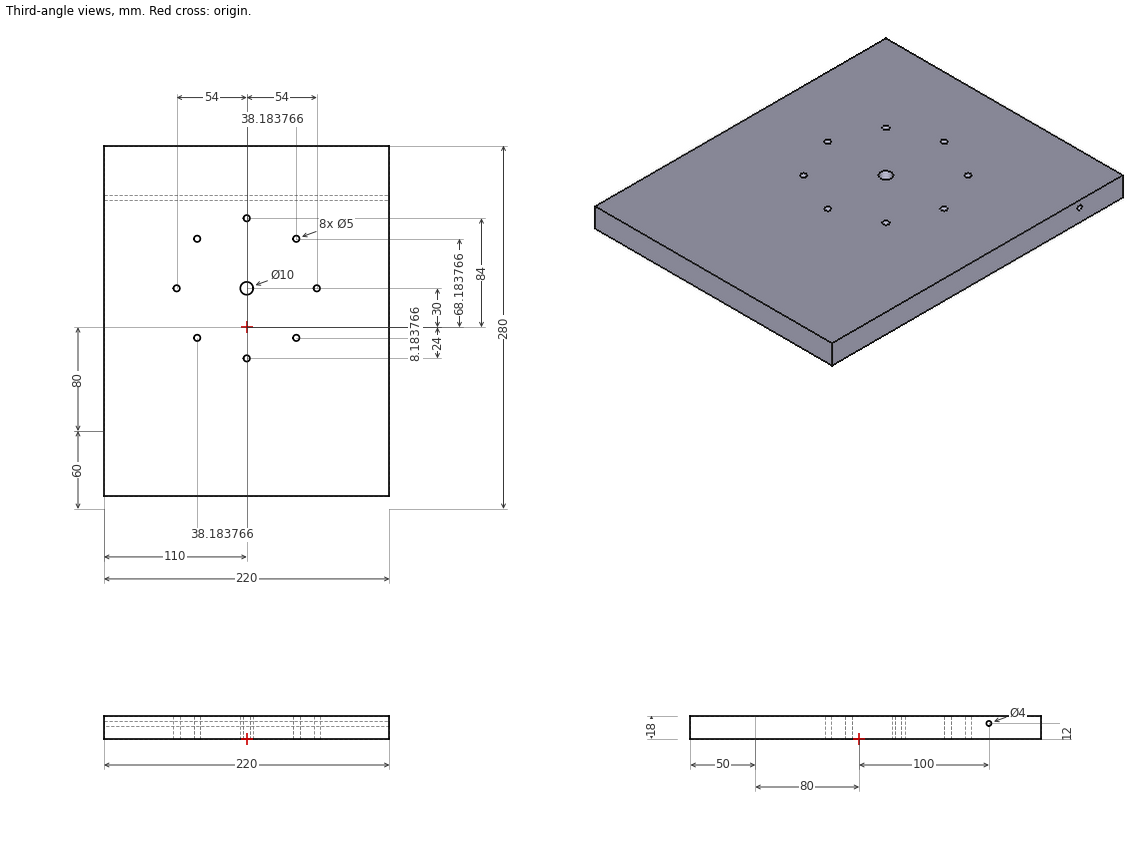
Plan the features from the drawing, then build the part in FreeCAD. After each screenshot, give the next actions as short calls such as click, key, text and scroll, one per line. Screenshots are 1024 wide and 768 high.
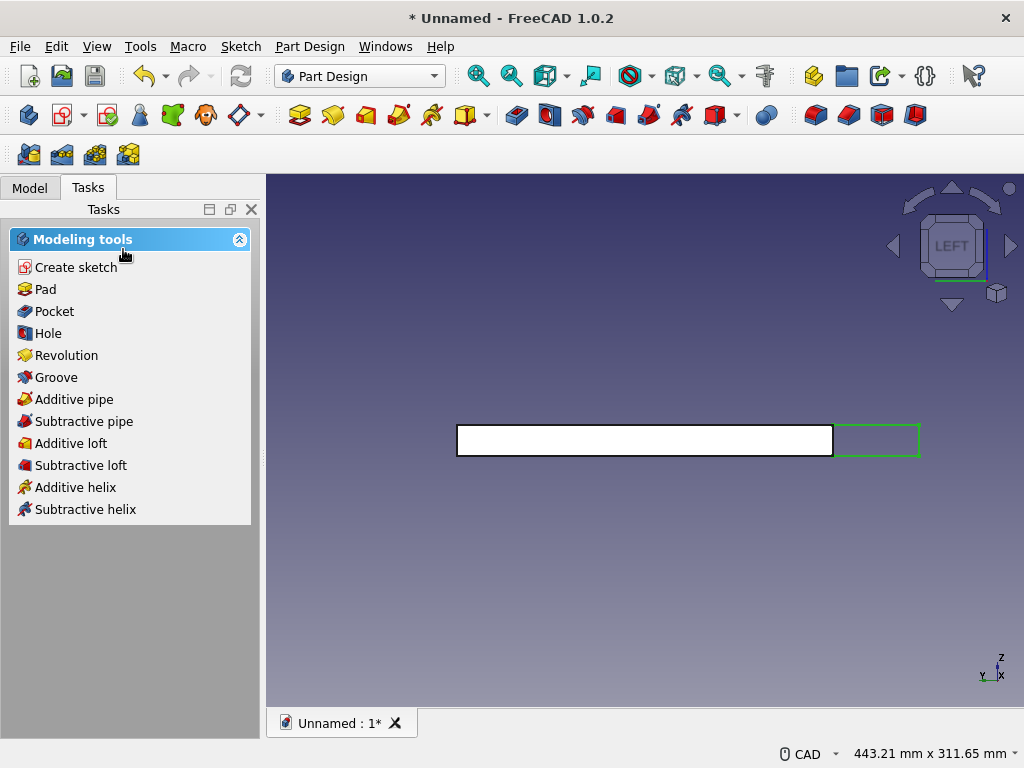
click(300, 116)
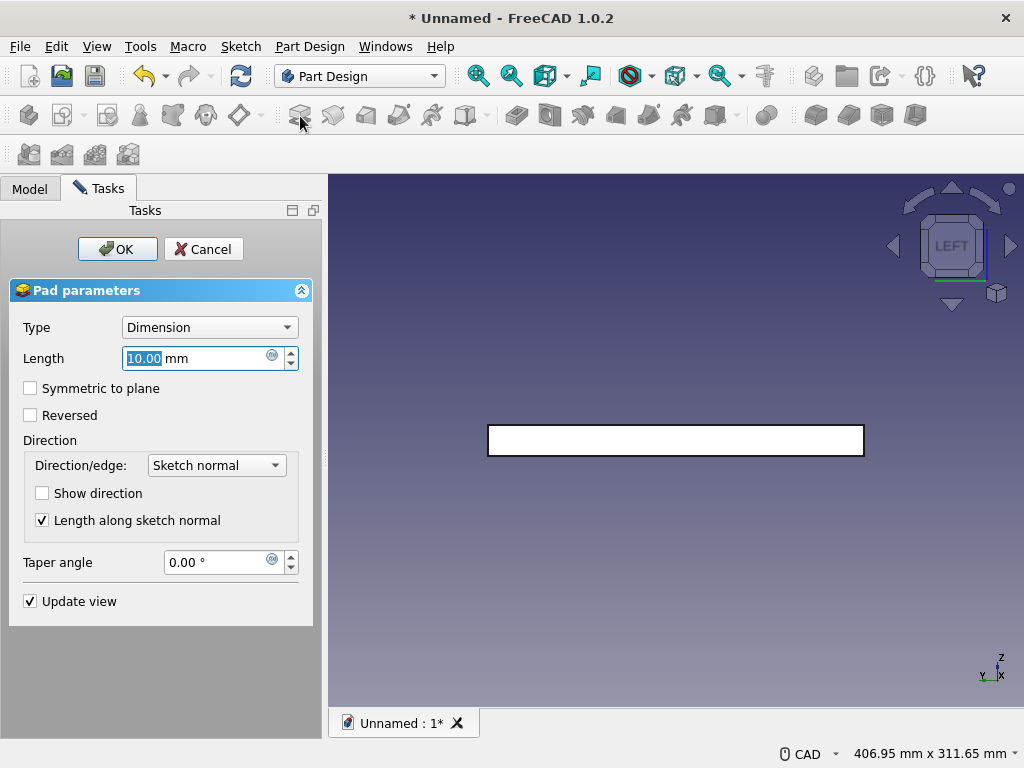
text(220)
key(Tab)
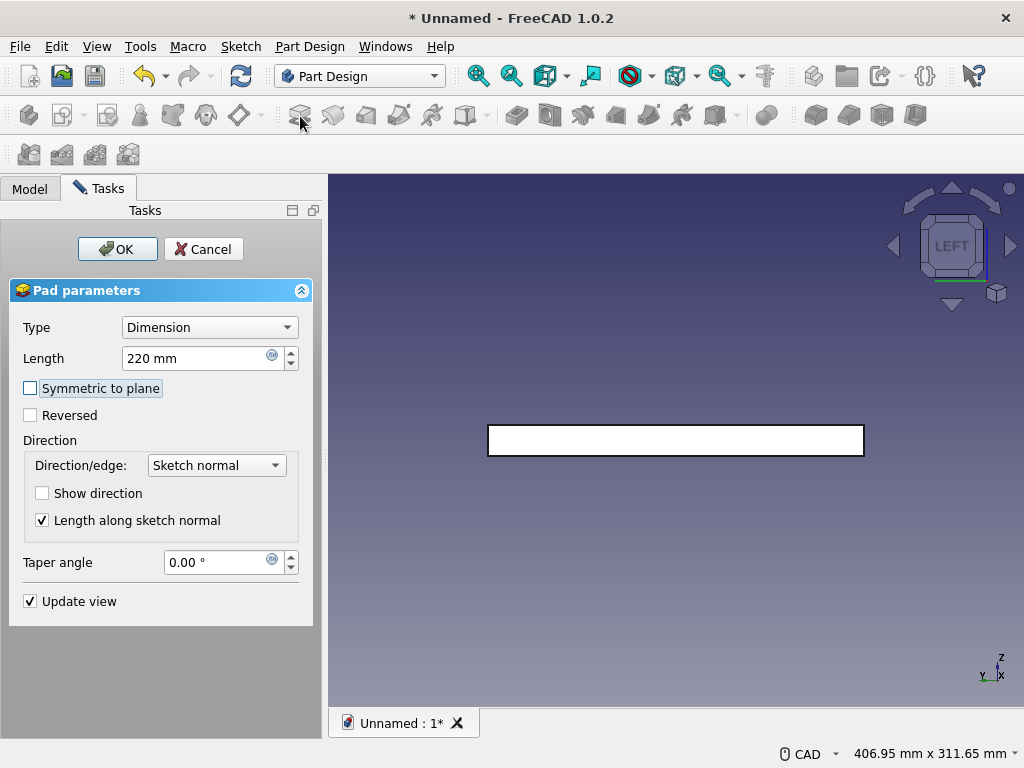
click(31, 415)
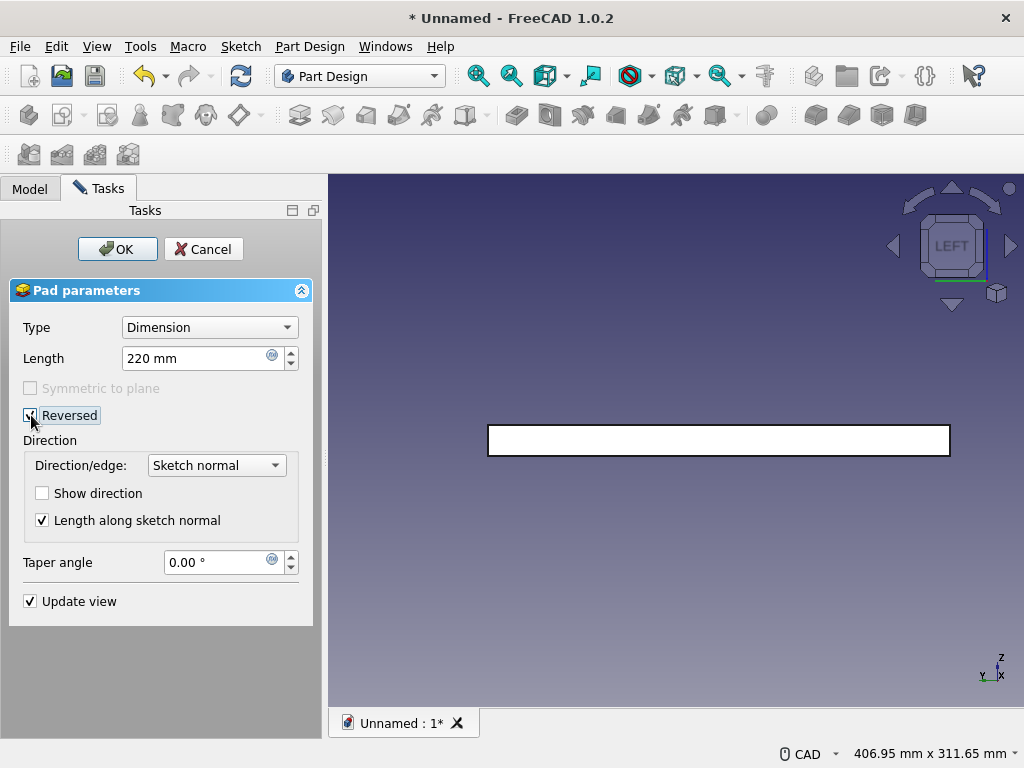
click(118, 249)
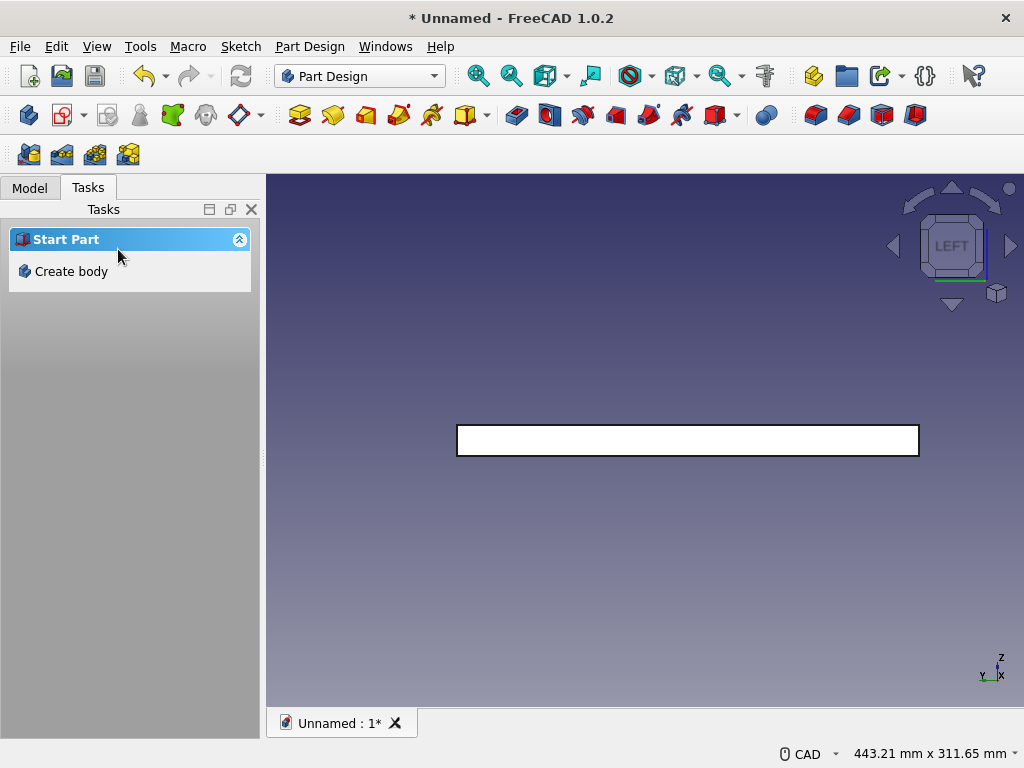
key(0)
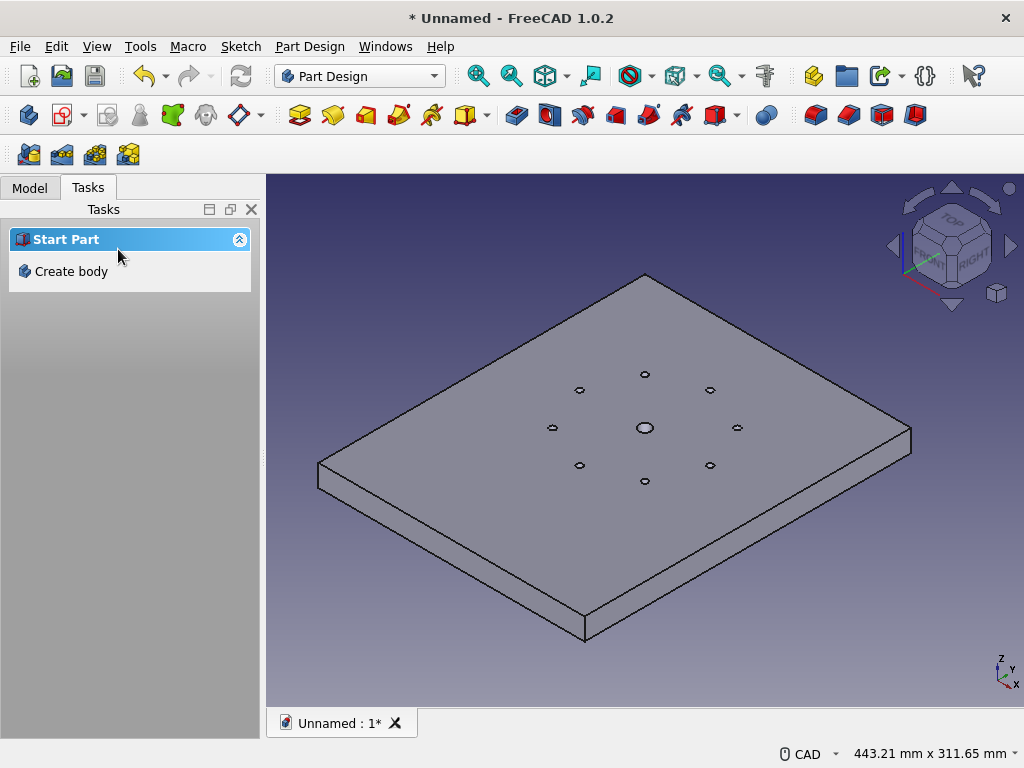
click(888, 453)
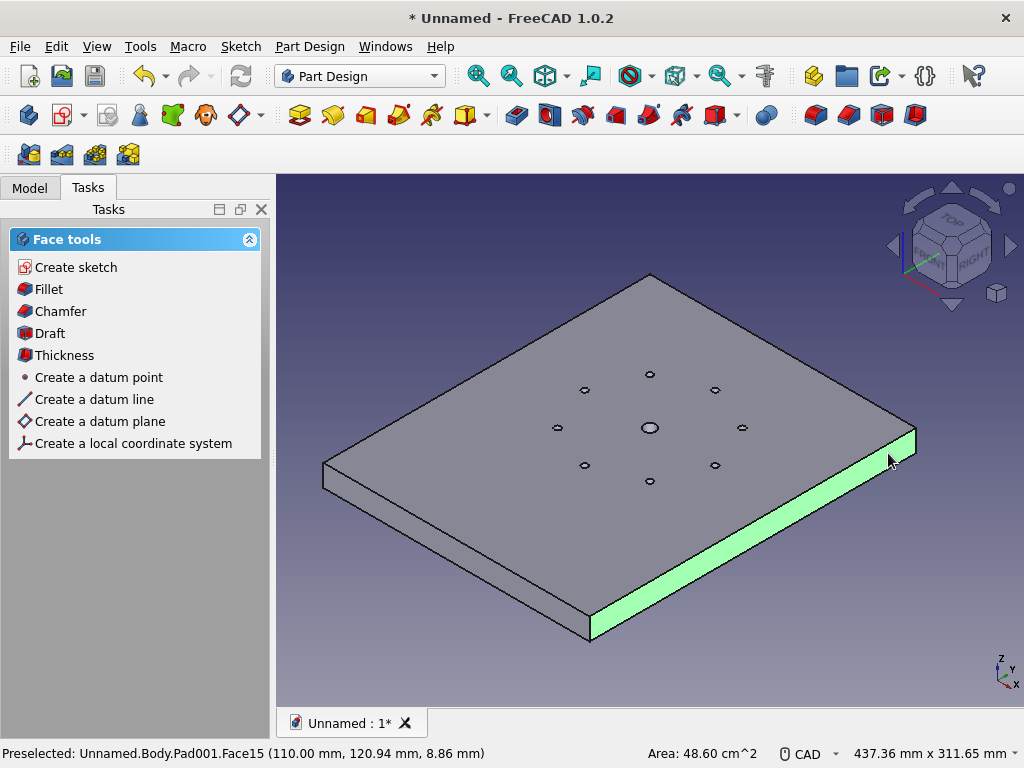
click(62, 116)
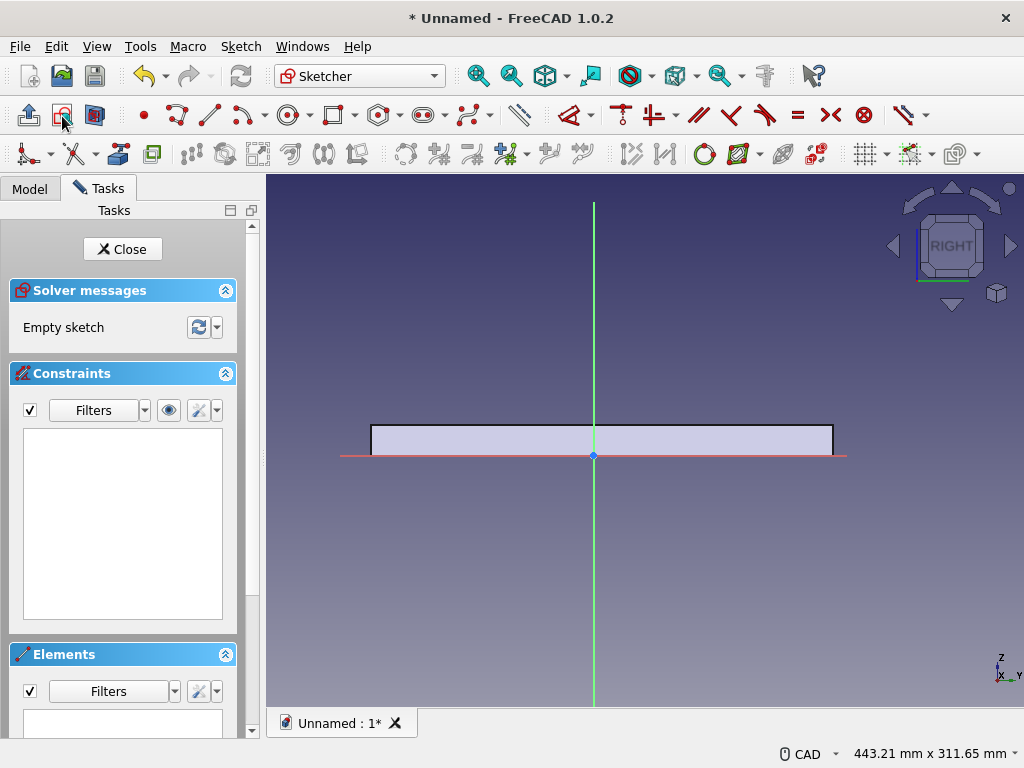
scroll(775, 435, up, 15)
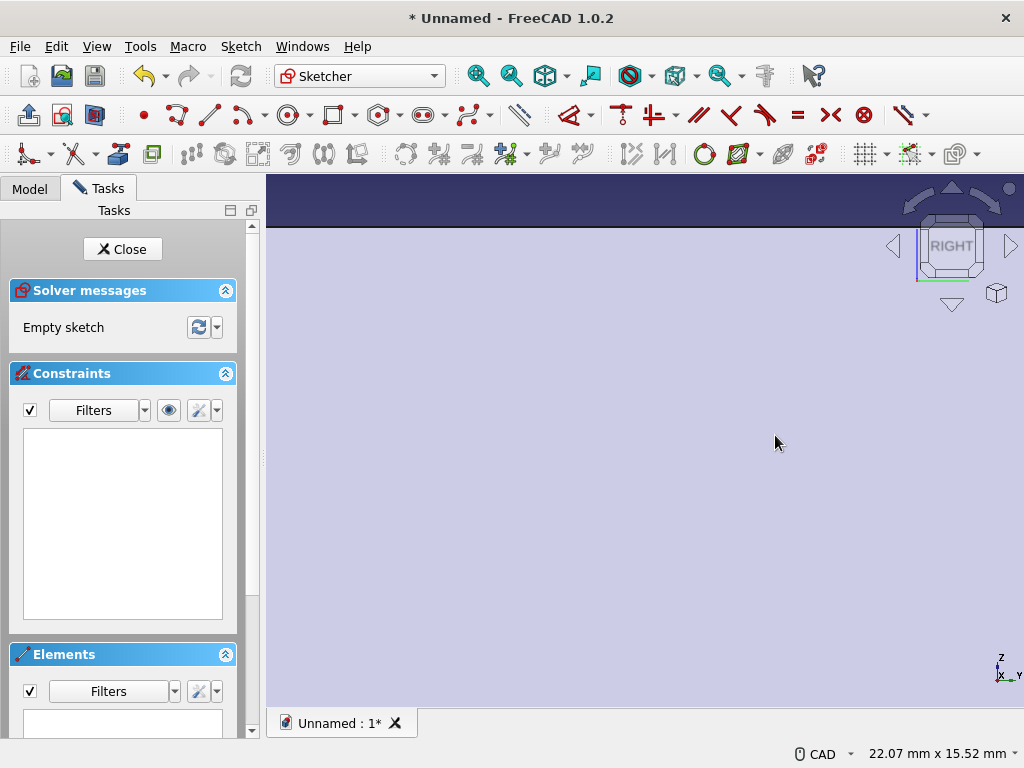
scroll(539, 427, up, 4)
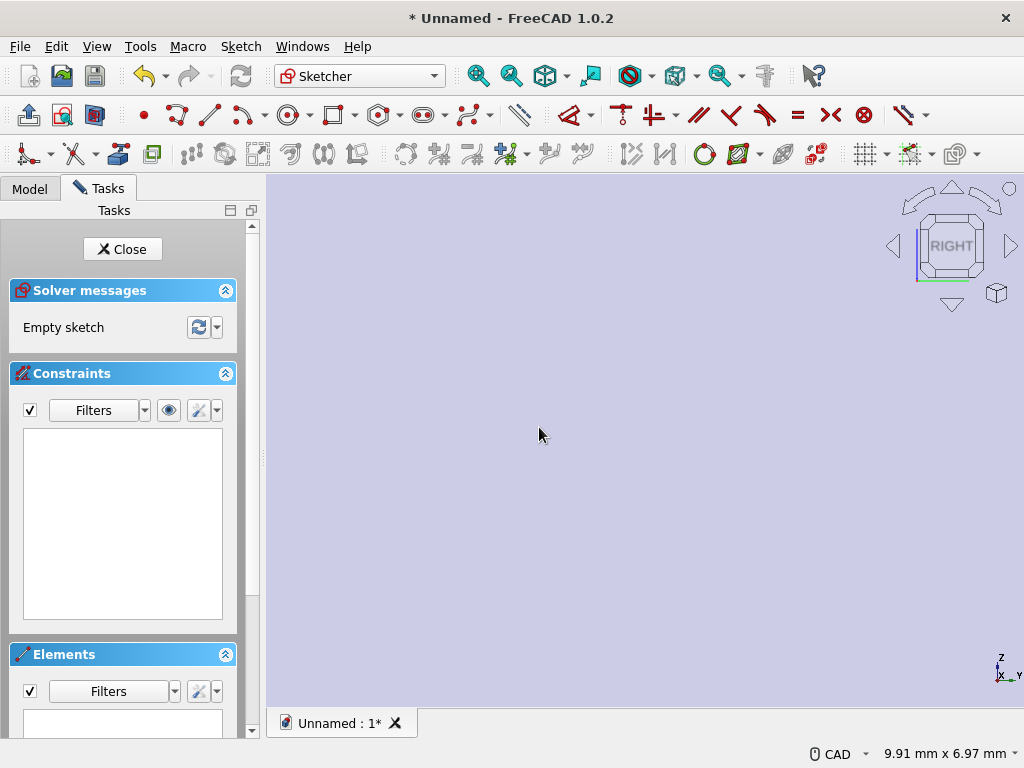
click(288, 116)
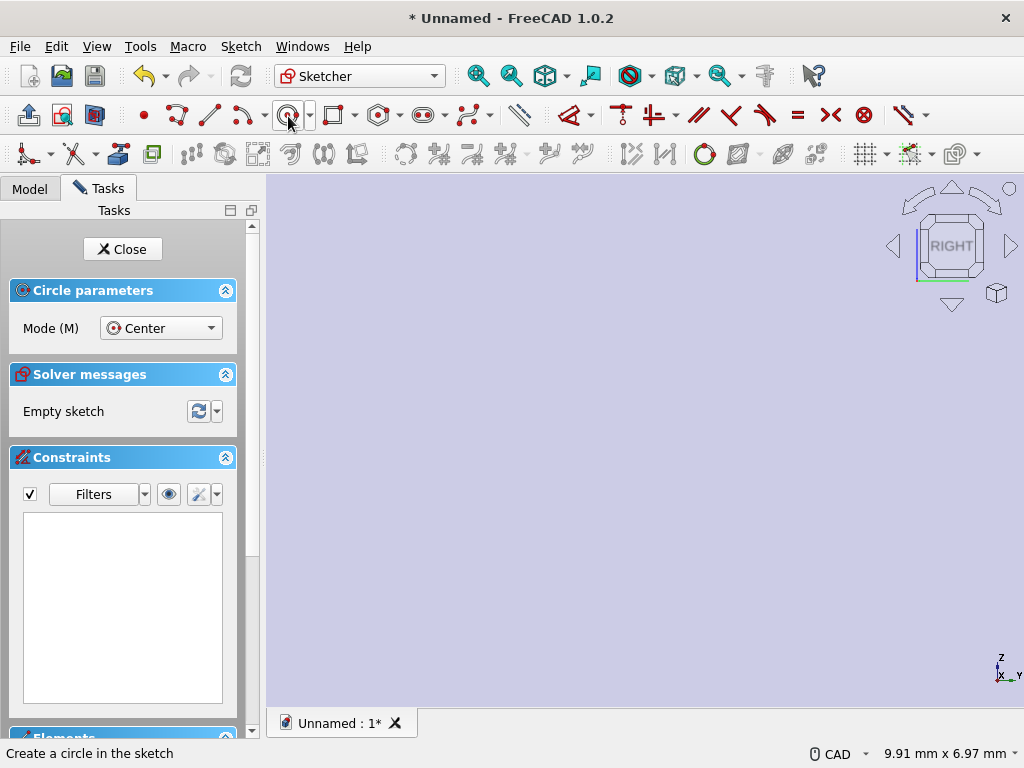
click(576, 440)
click(684, 332)
key(Escape)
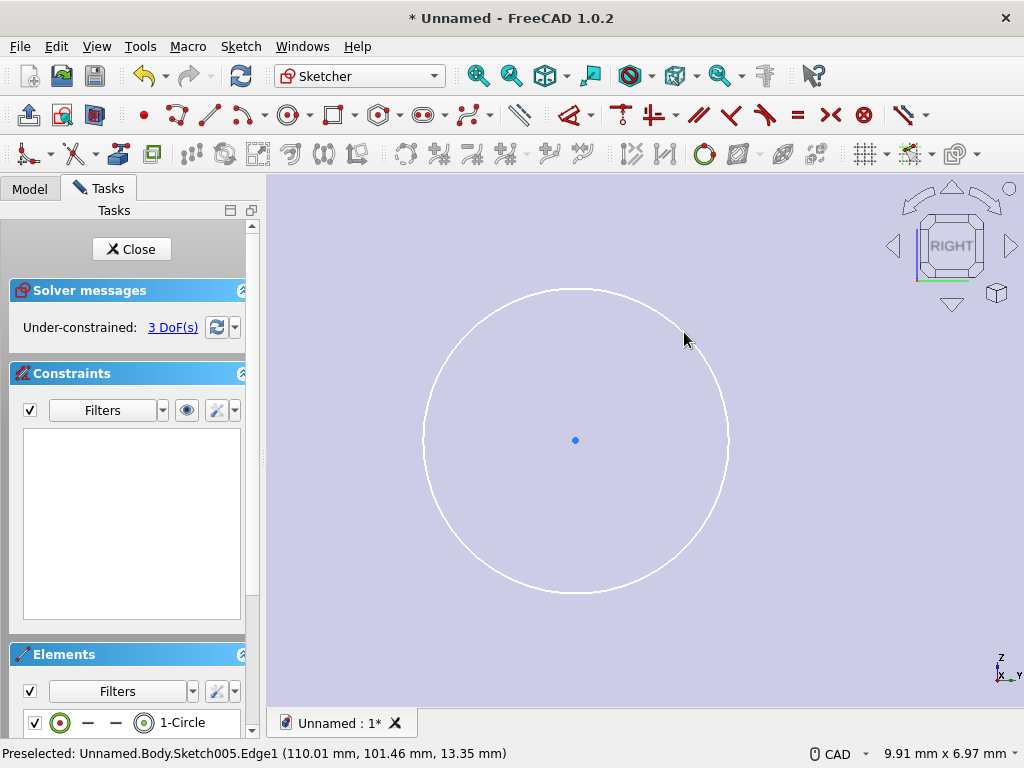
key(d)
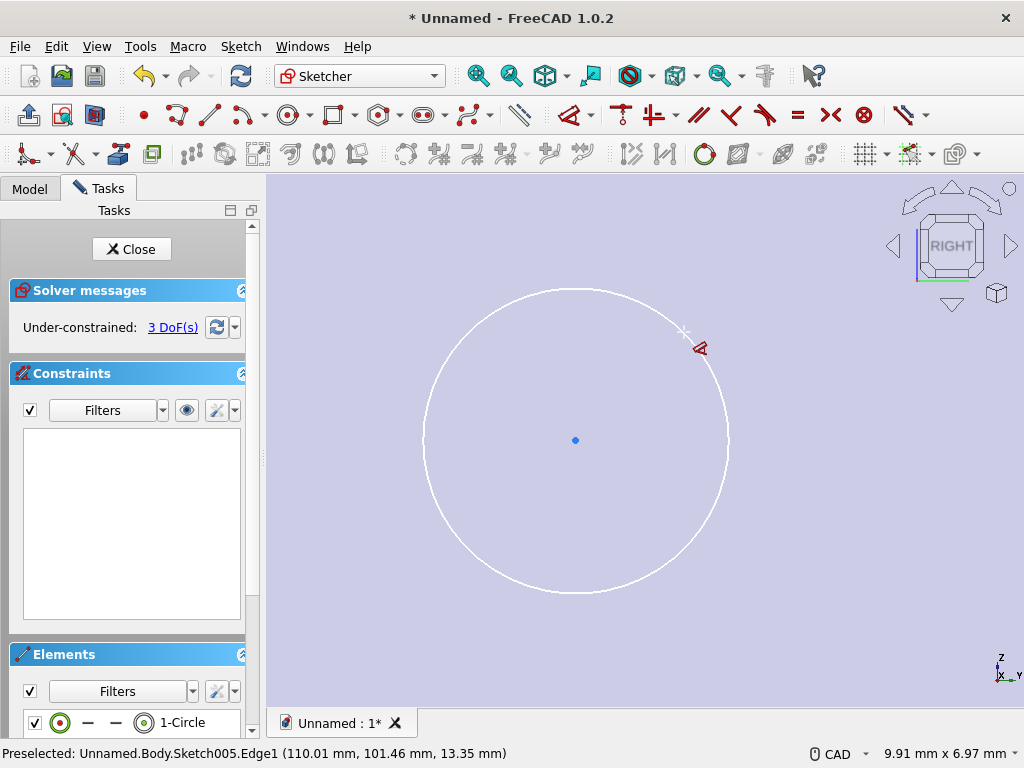
click(684, 333)
click(707, 310)